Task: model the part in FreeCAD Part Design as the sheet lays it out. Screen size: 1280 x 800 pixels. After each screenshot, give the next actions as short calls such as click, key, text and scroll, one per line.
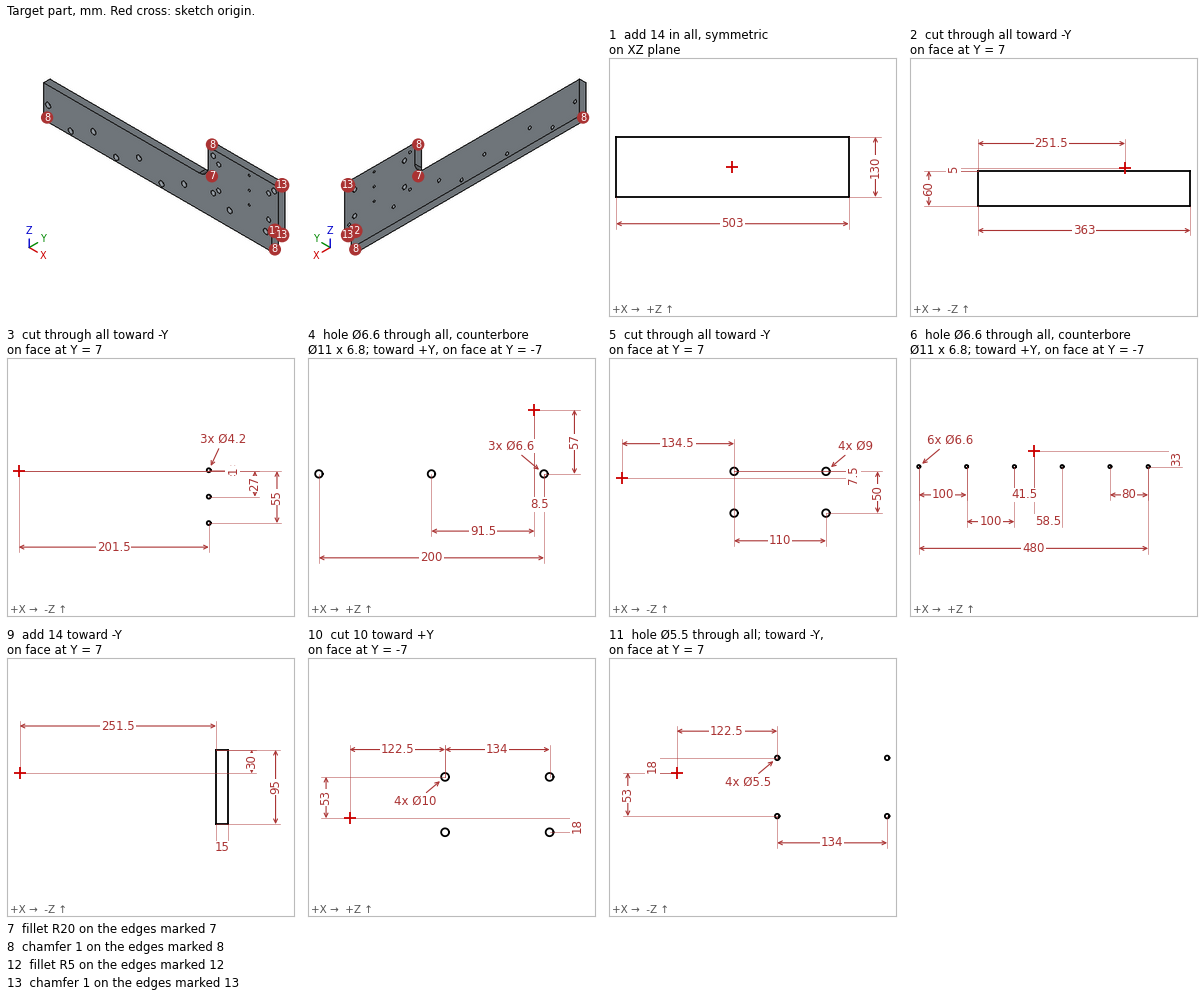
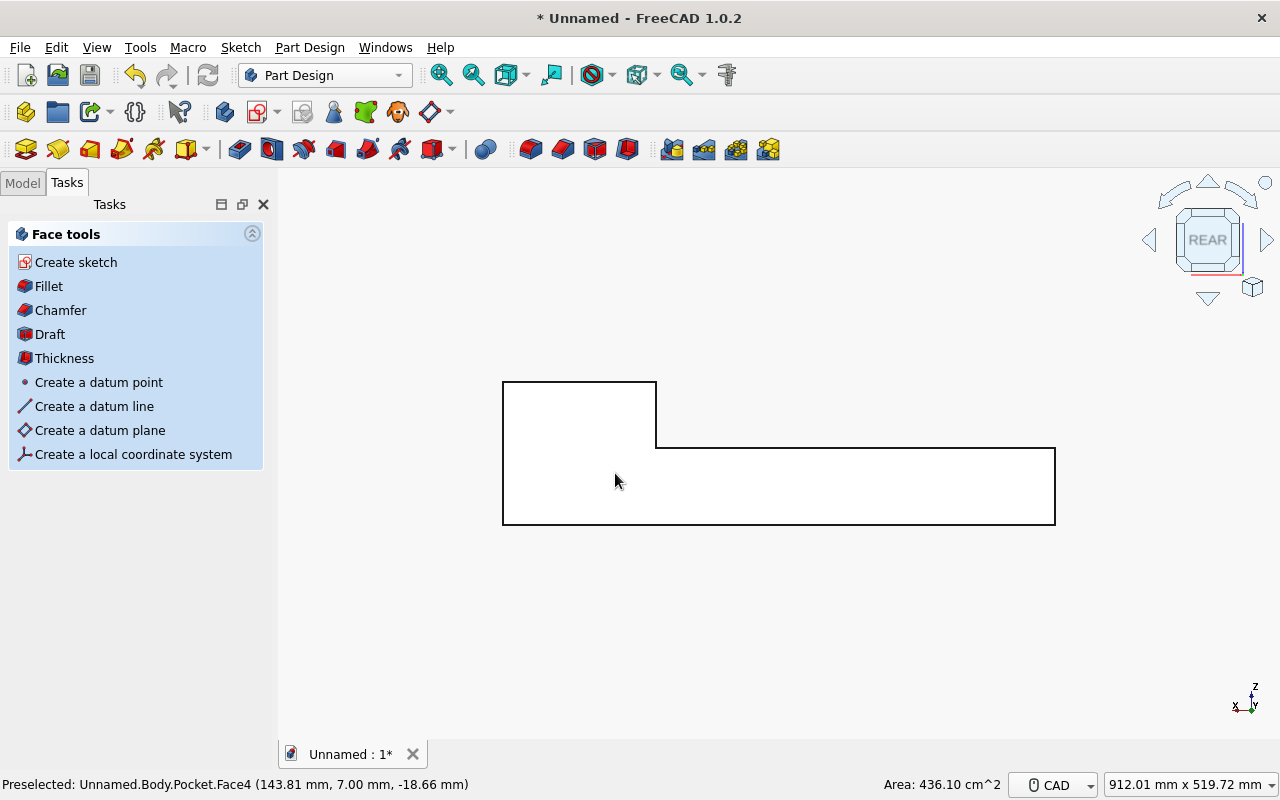
click(258, 112)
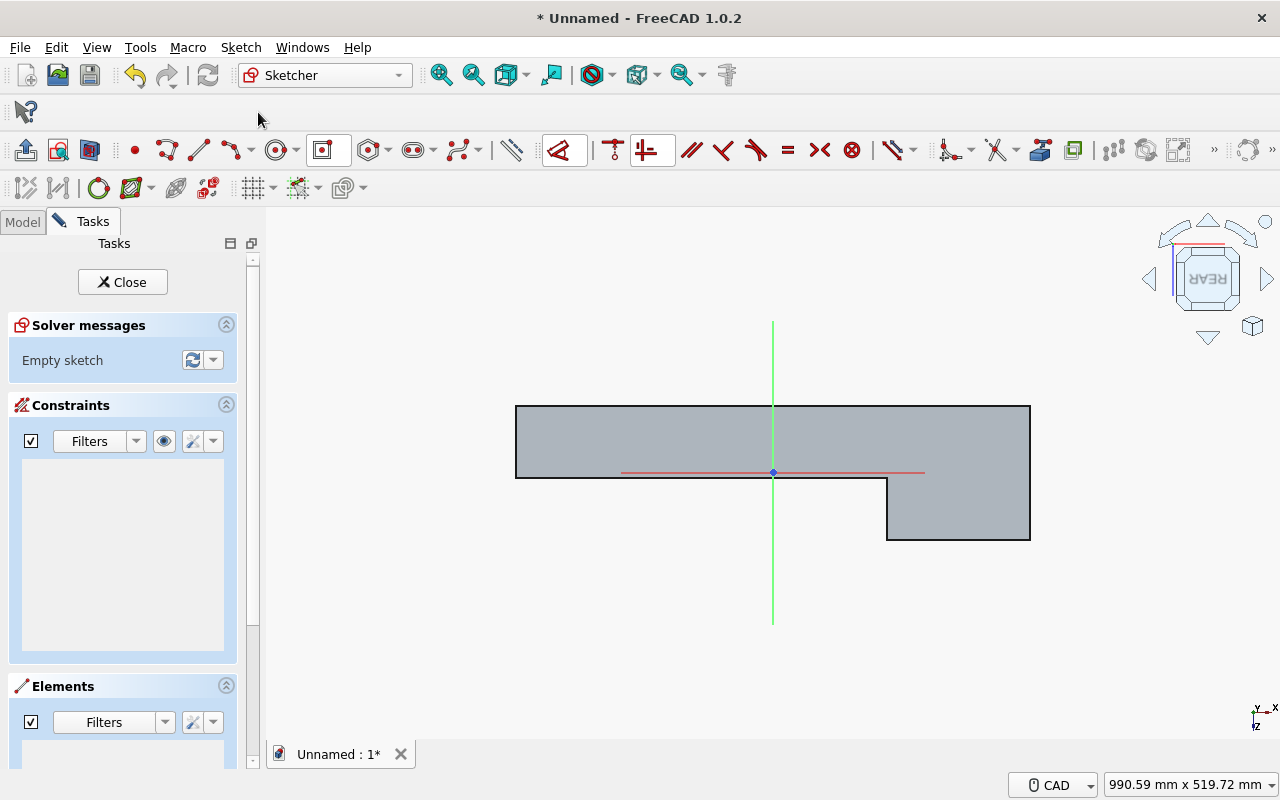
scroll(1049, 508, up, 8)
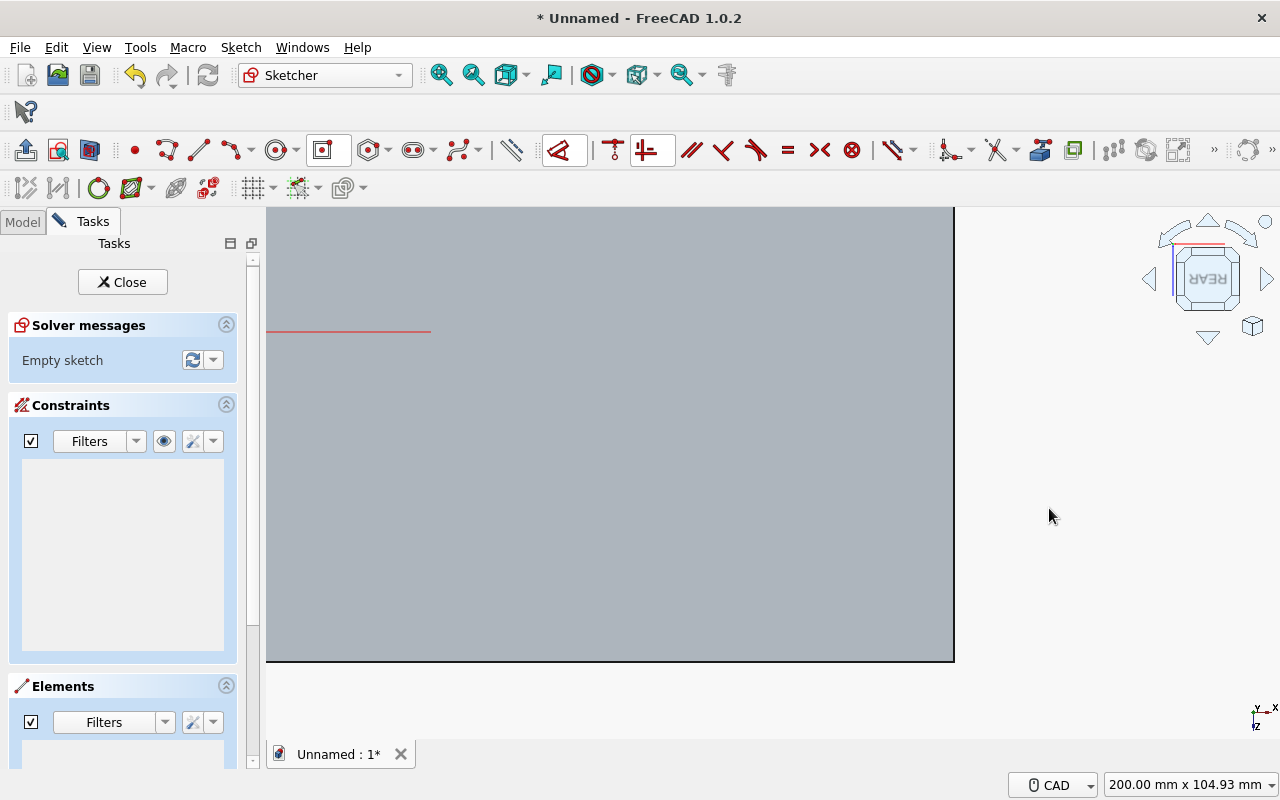
click(276, 150)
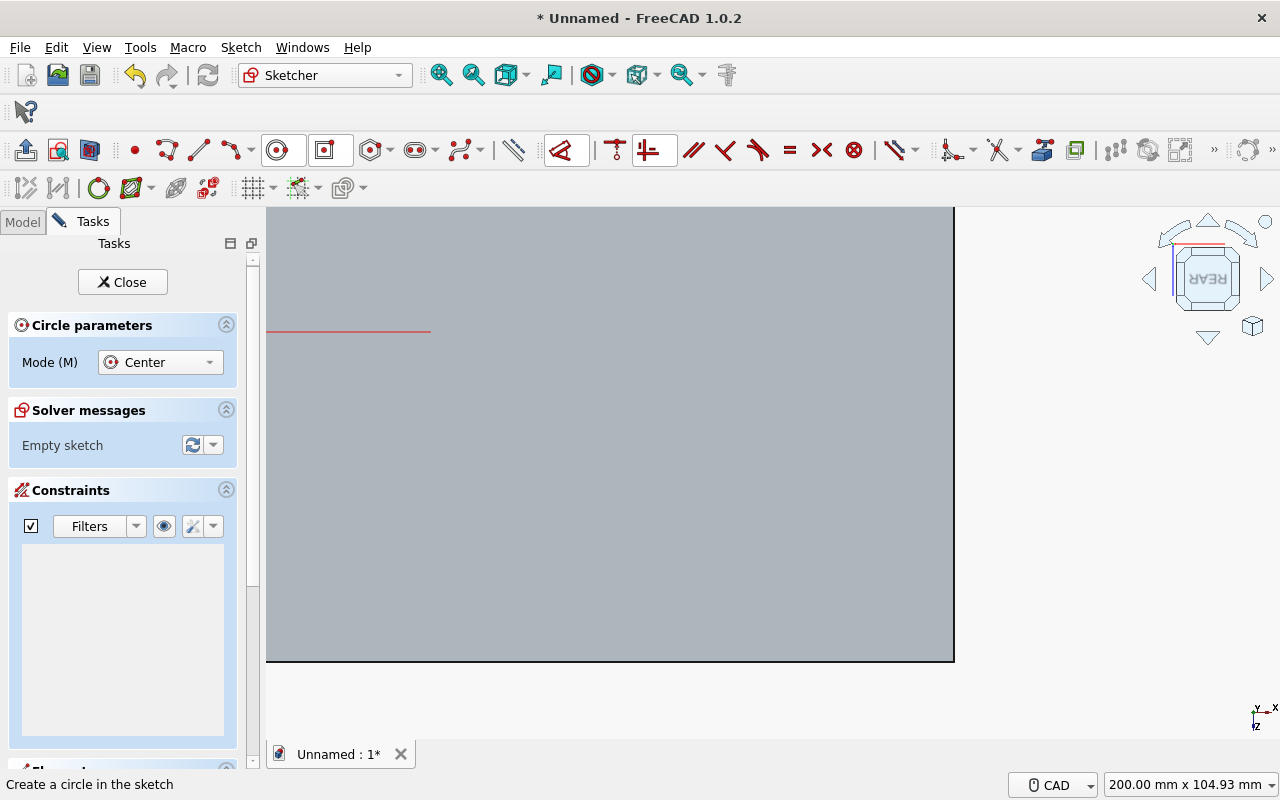
scroll(701, 611, up, 4)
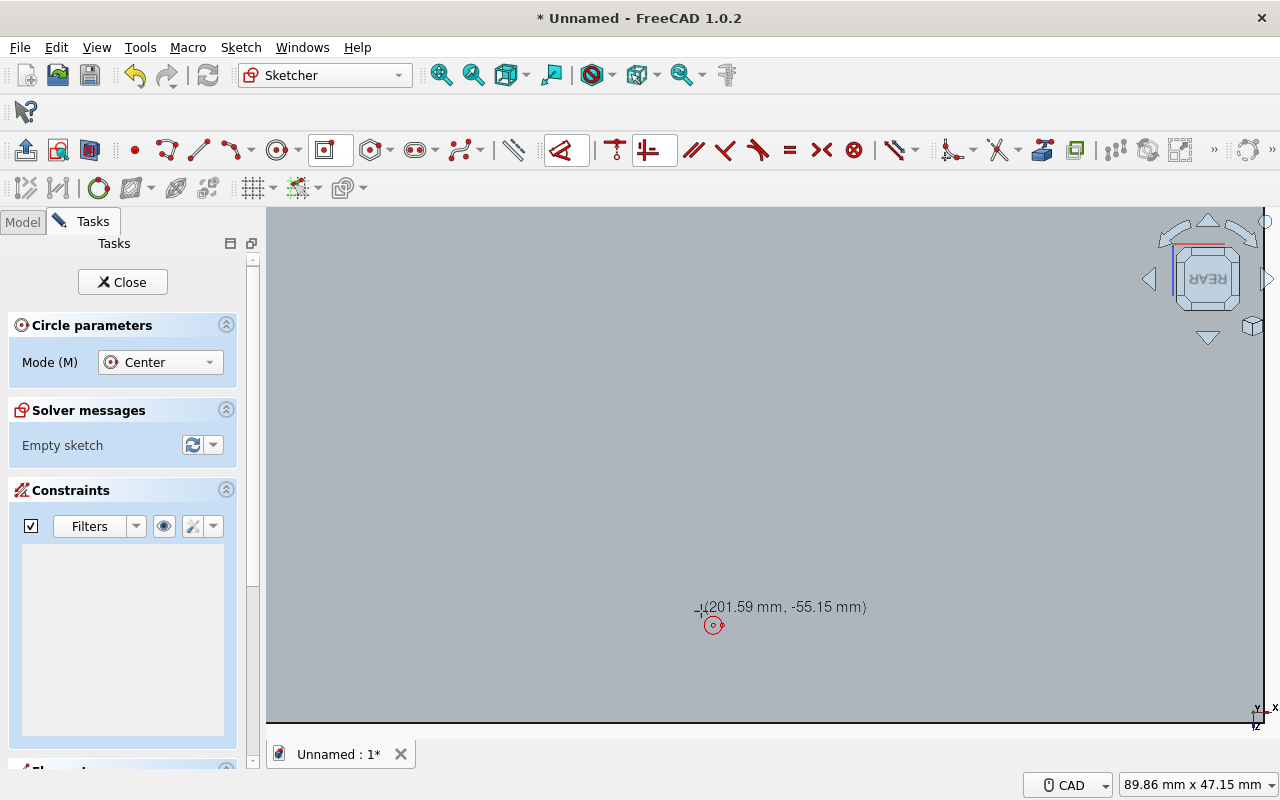
click(699, 611)
click(716, 594)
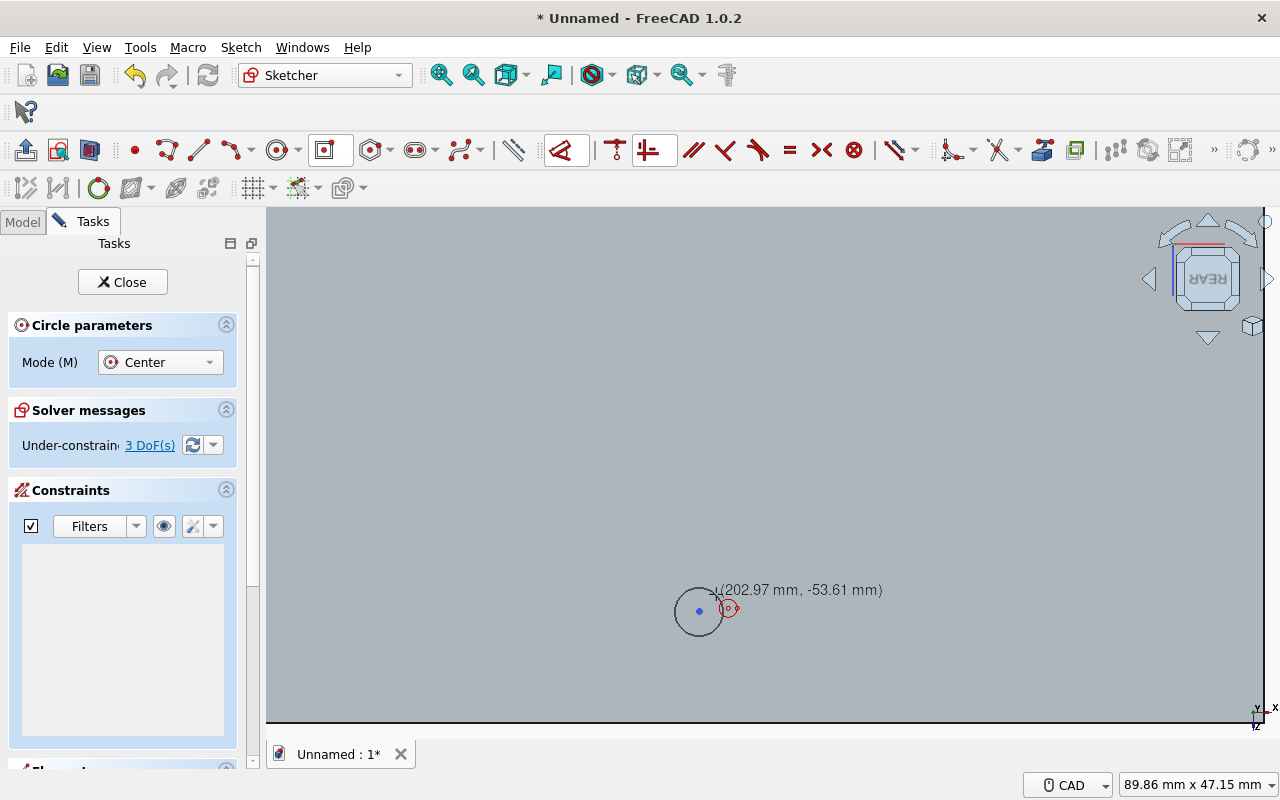
click(699, 295)
click(716, 278)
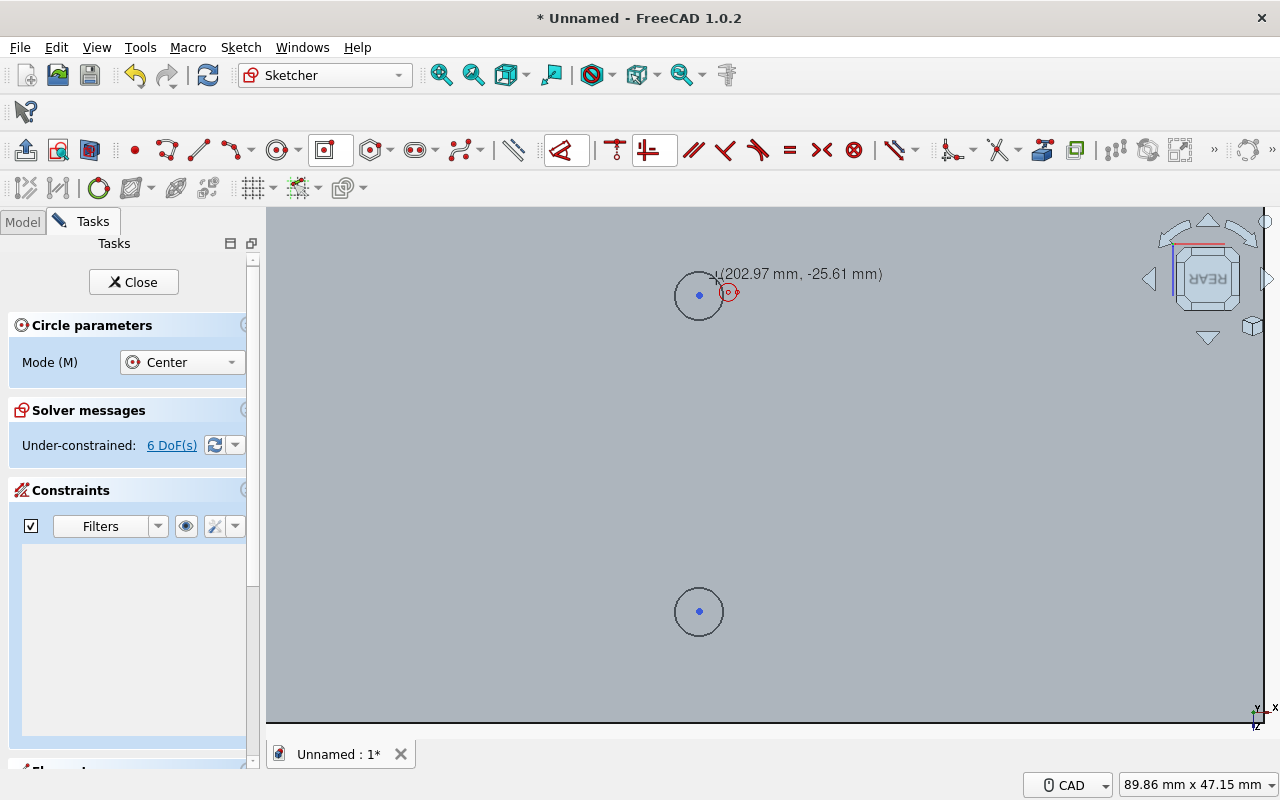
scroll(709, 618, down, 4)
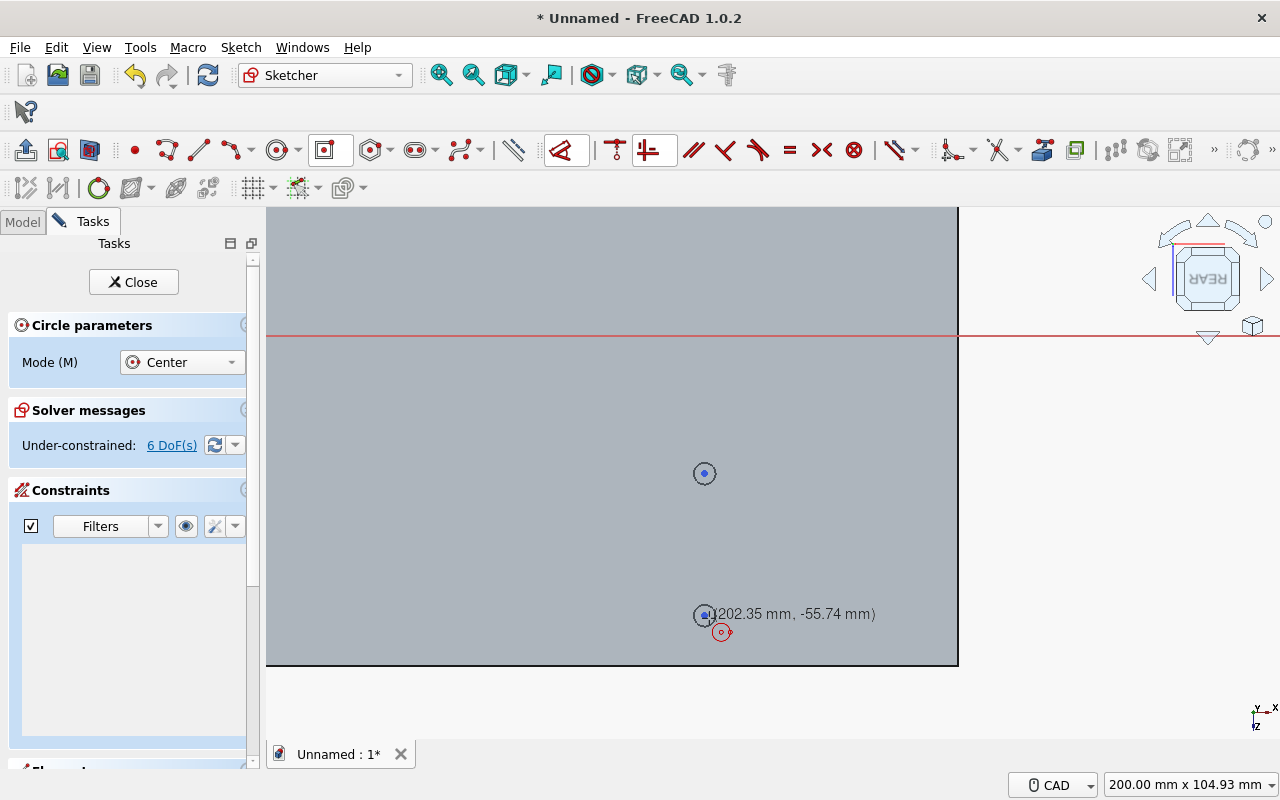
scroll(705, 331, up, 6)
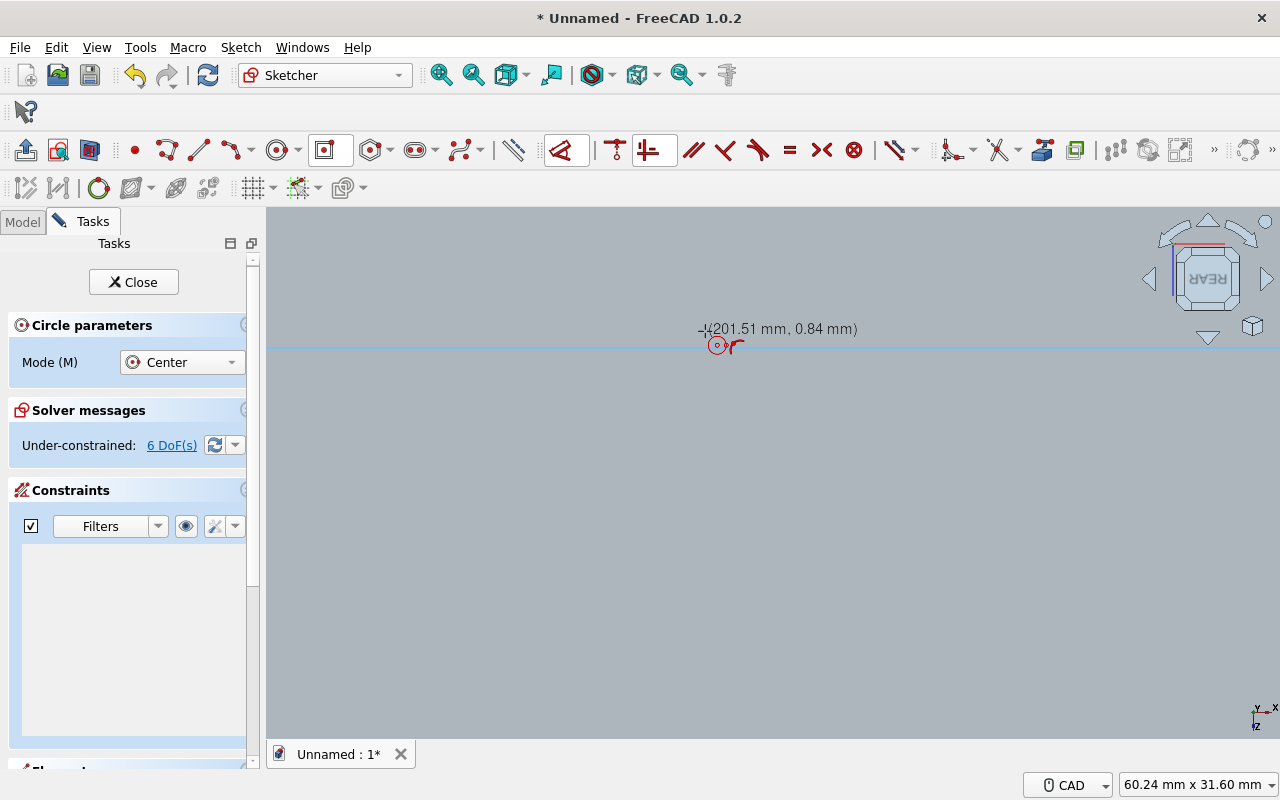
click(704, 331)
click(729, 306)
key(Escape)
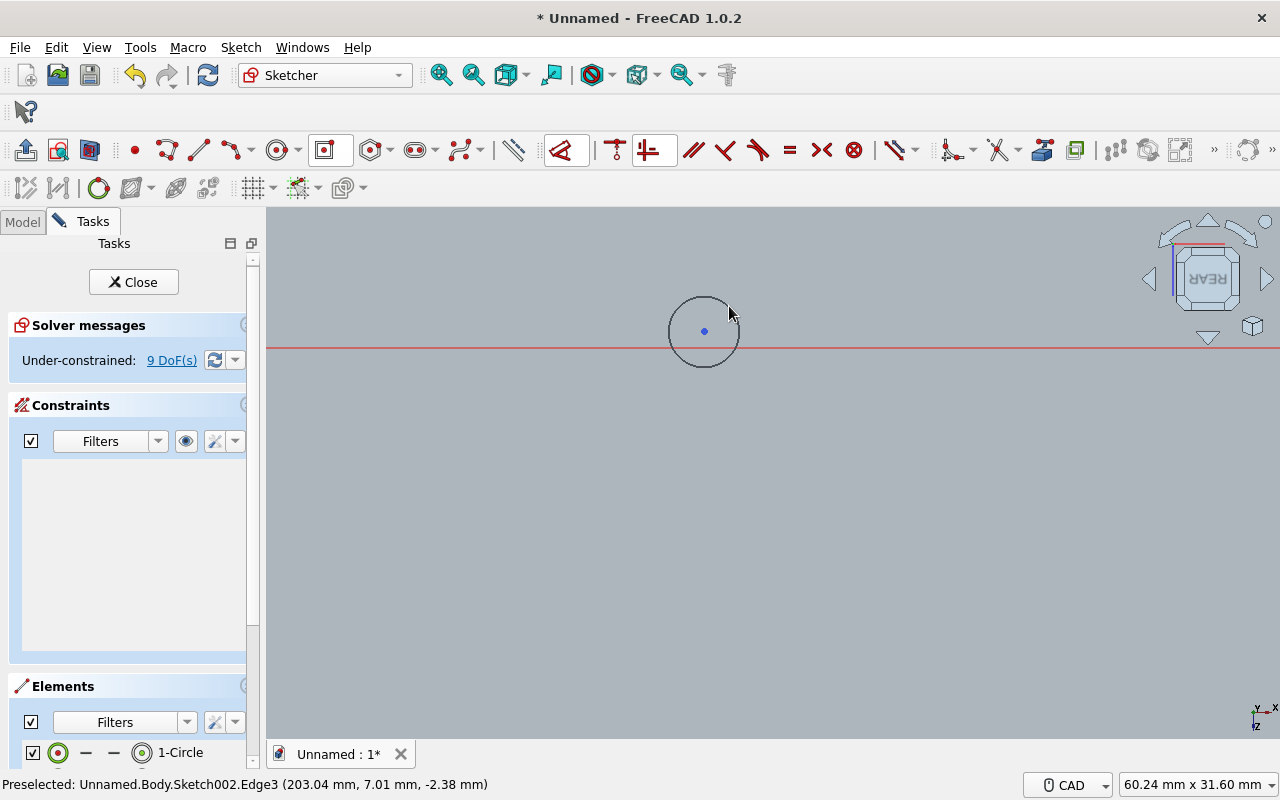
scroll(705, 331, down, 6)